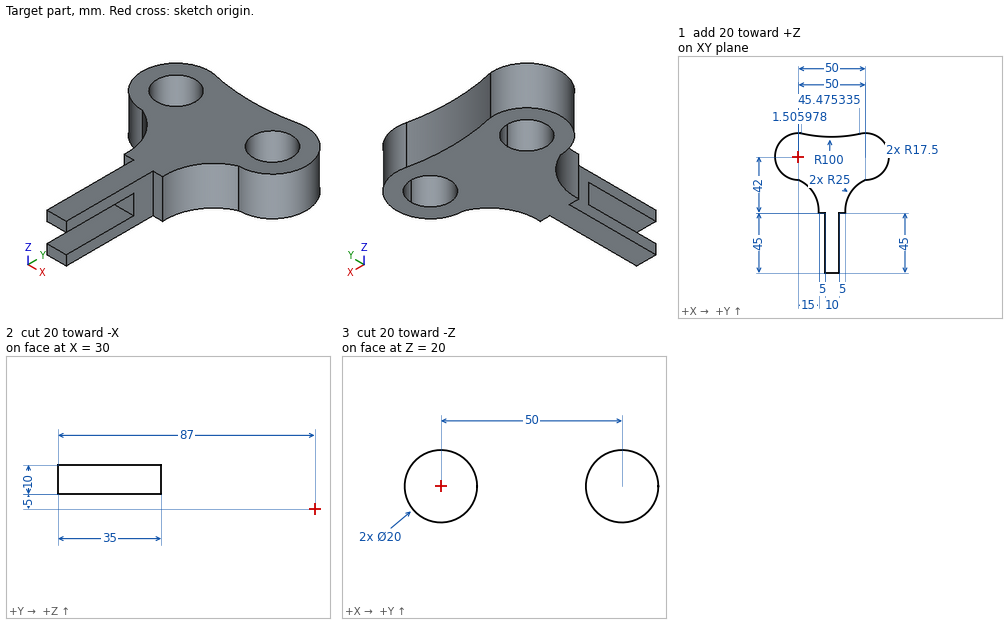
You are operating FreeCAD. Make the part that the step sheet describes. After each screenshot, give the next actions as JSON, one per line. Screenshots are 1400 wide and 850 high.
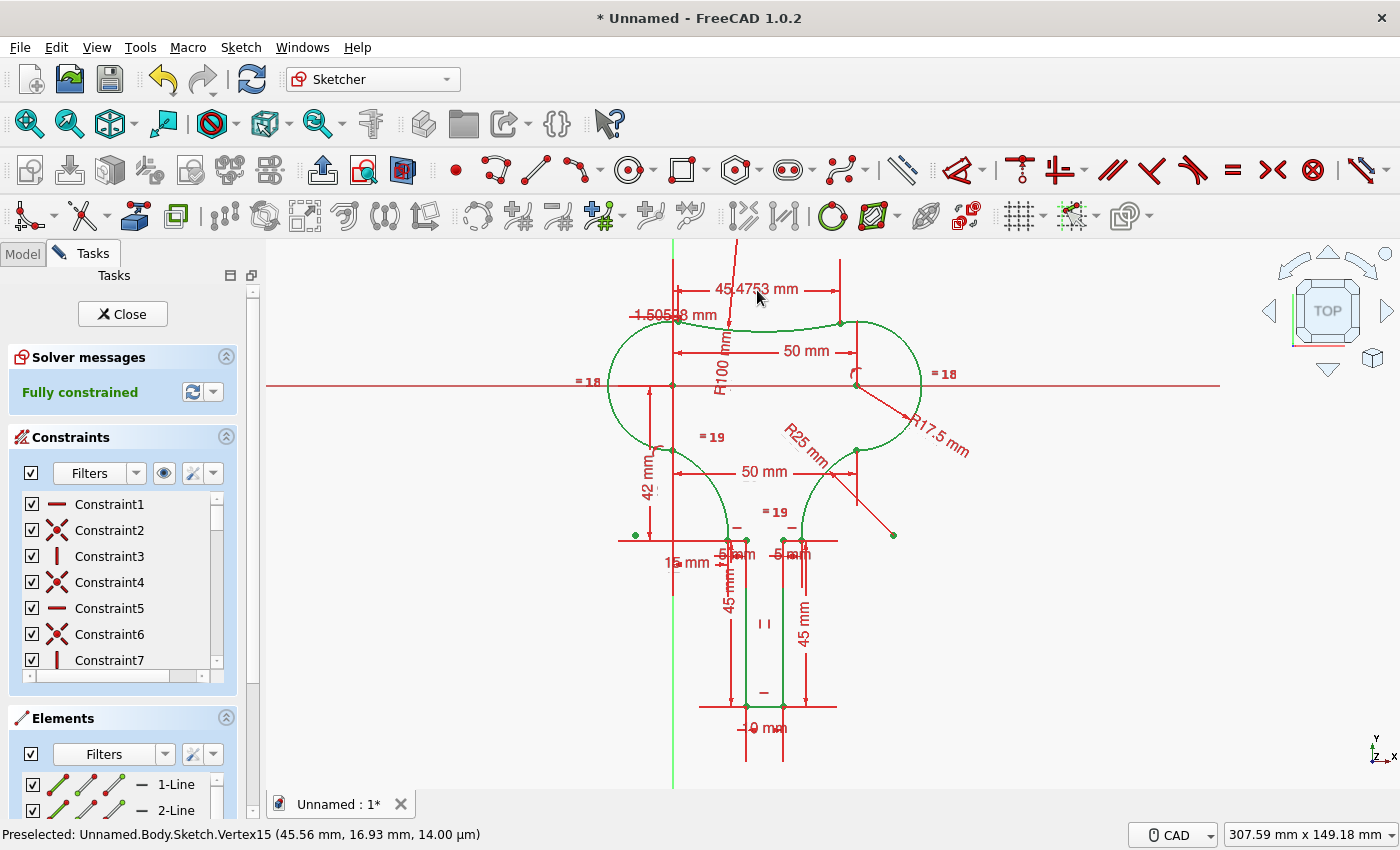
{"action": "left_click", "coordinate": [123, 314]}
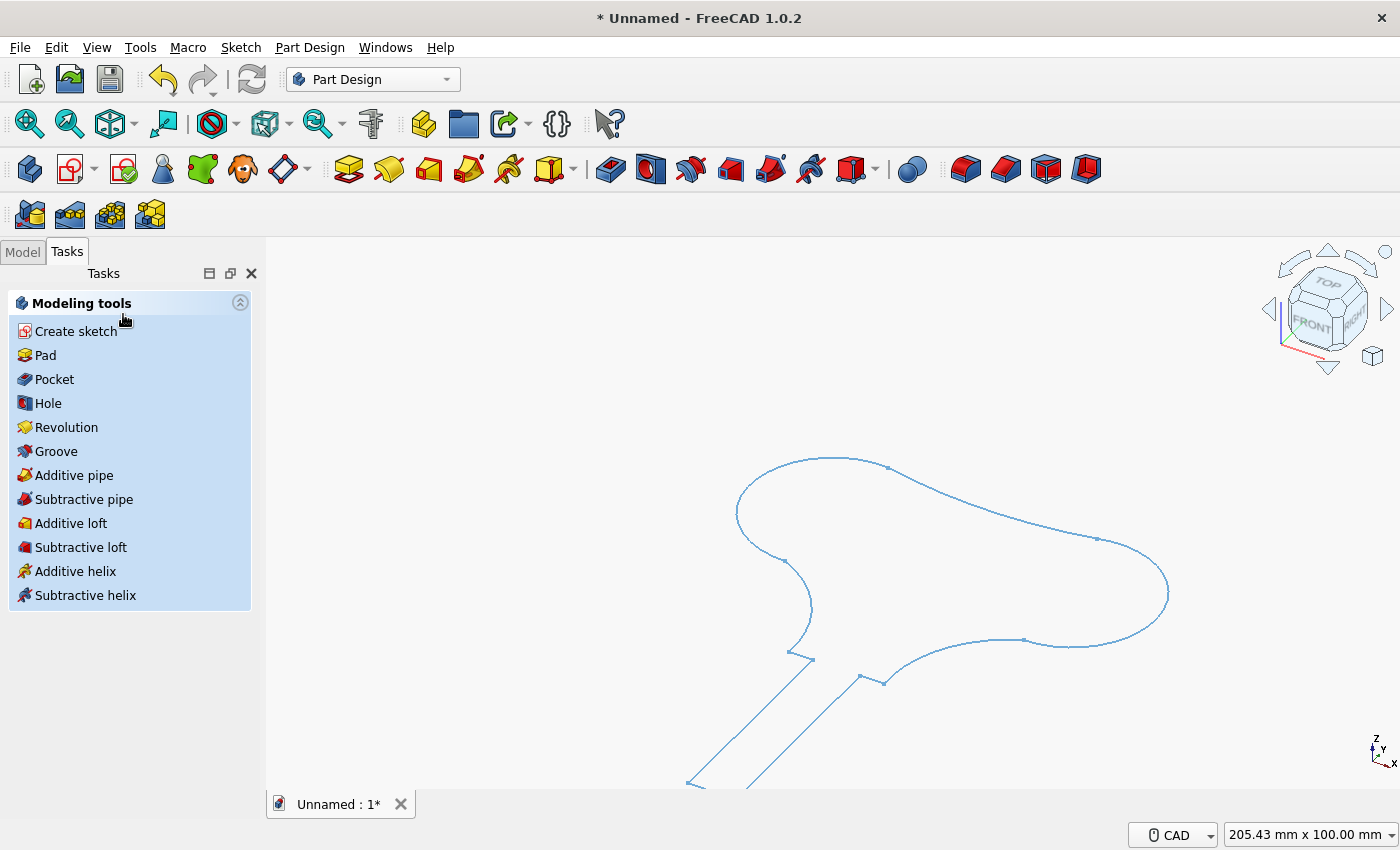
{"action": "left_click", "coordinate": [350, 170]}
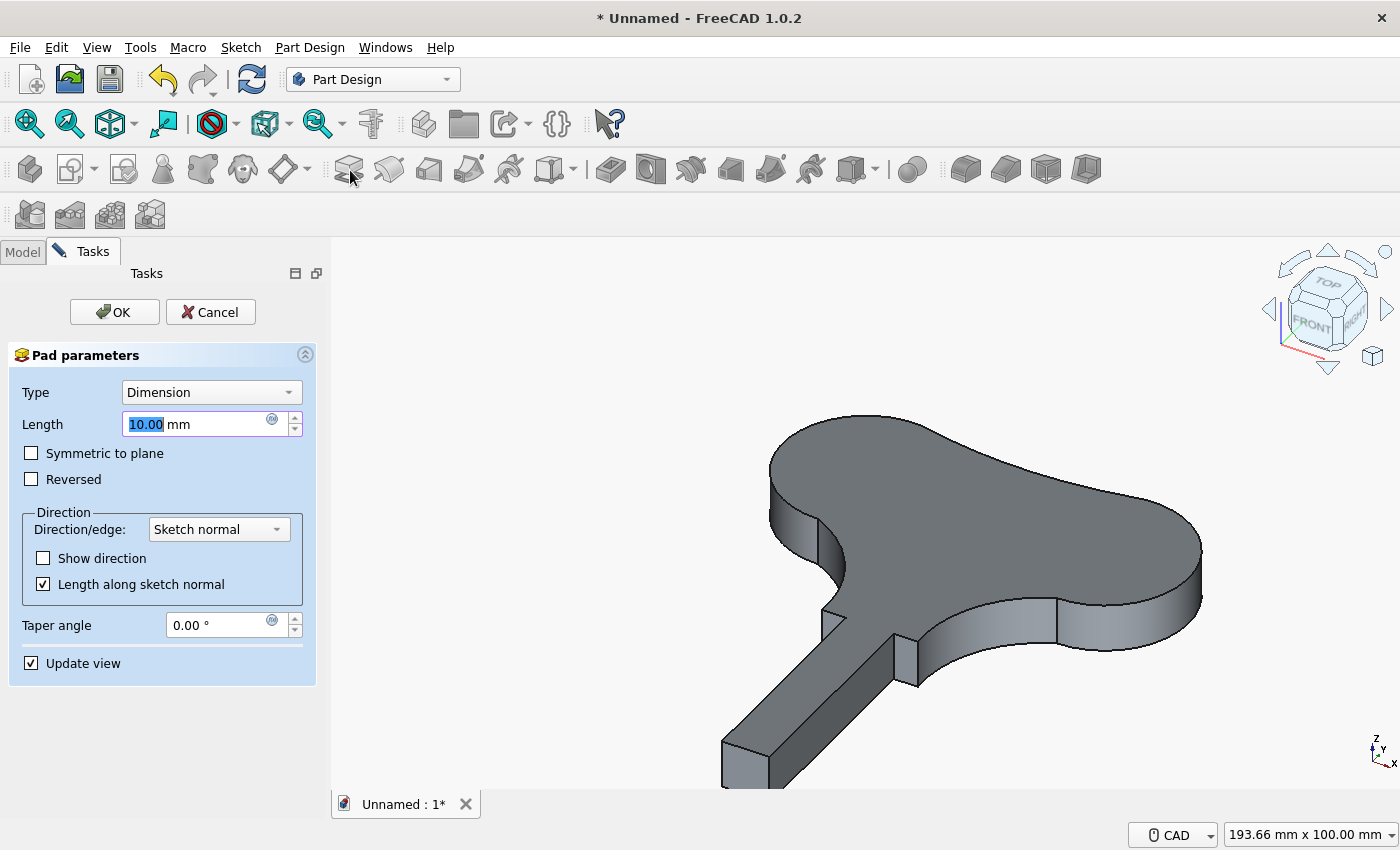
{"action": "type", "text": "20"}
{"action": "key", "text": "Tab"}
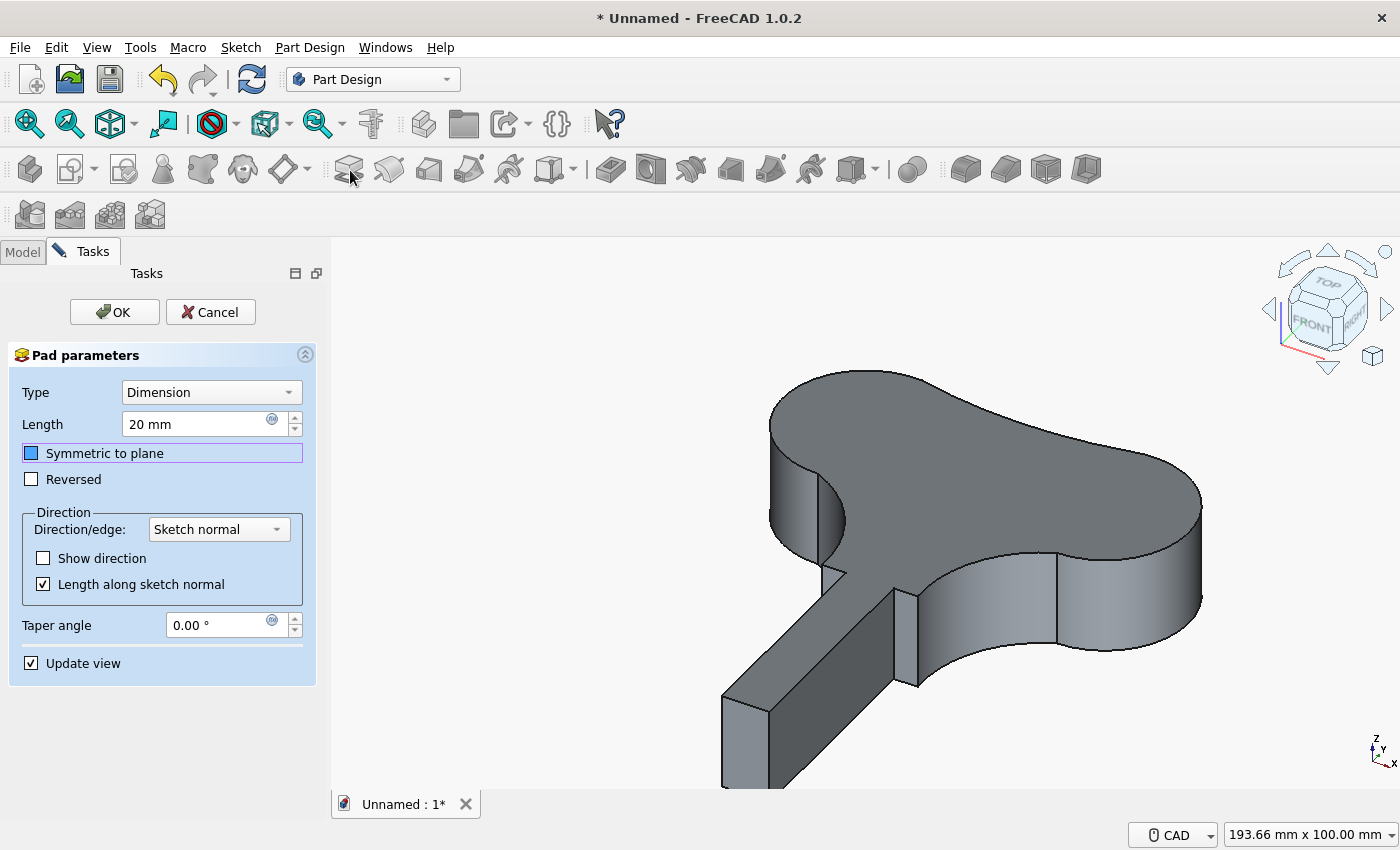
{"action": "left_click", "coordinate": [115, 312]}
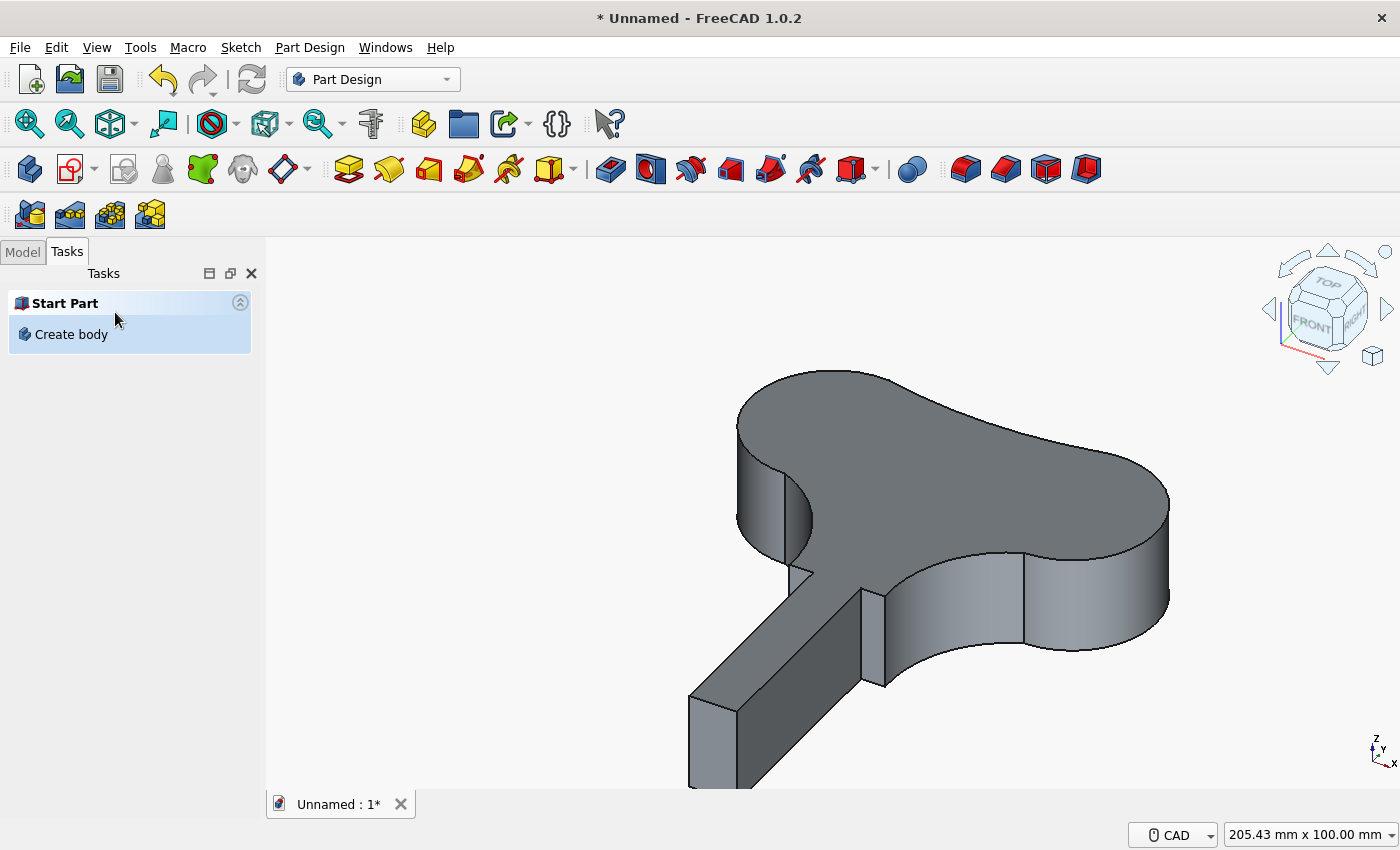
{"action": "left_click", "coordinate": [30, 124]}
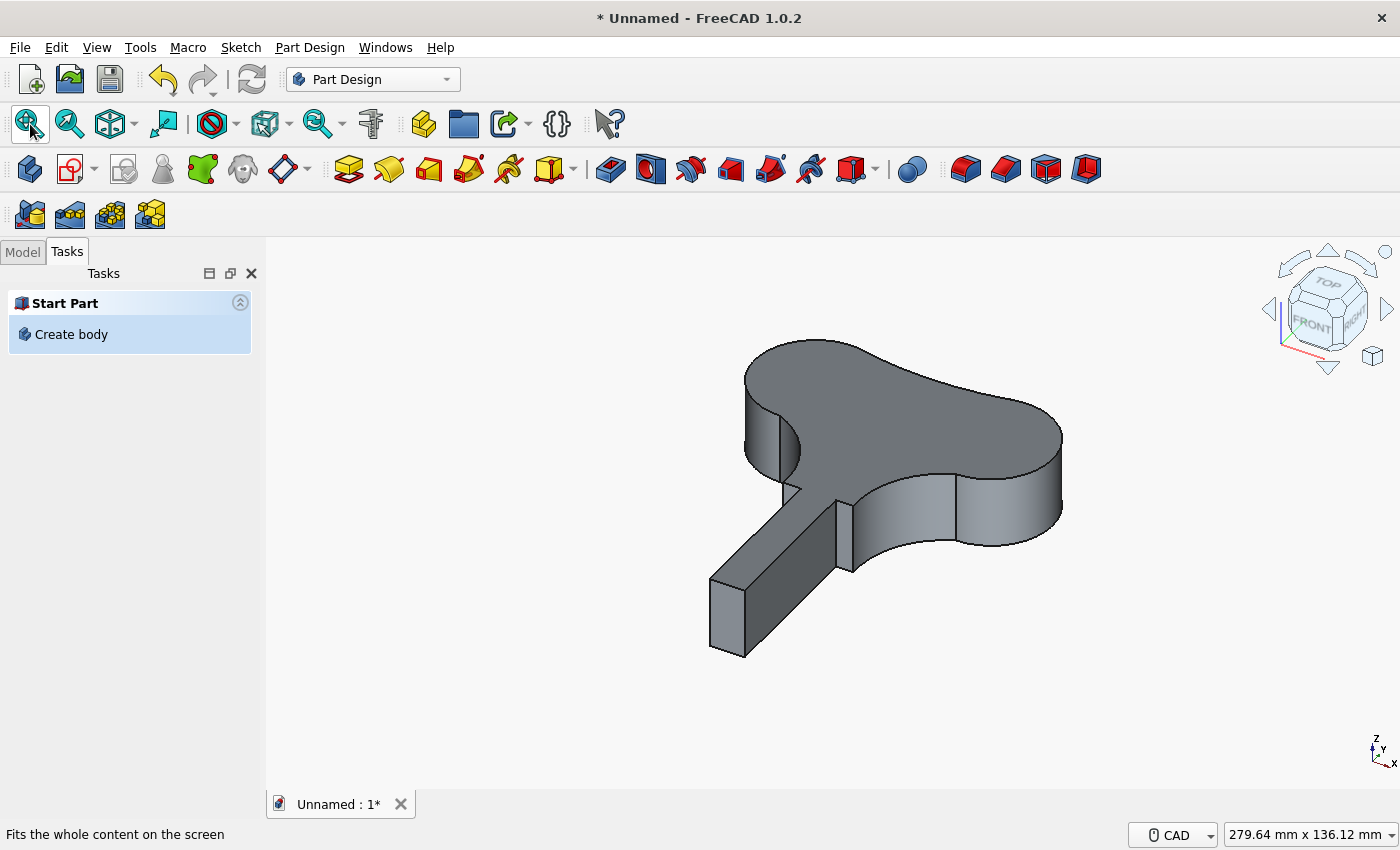
{"action": "left_click", "coordinate": [803, 565]}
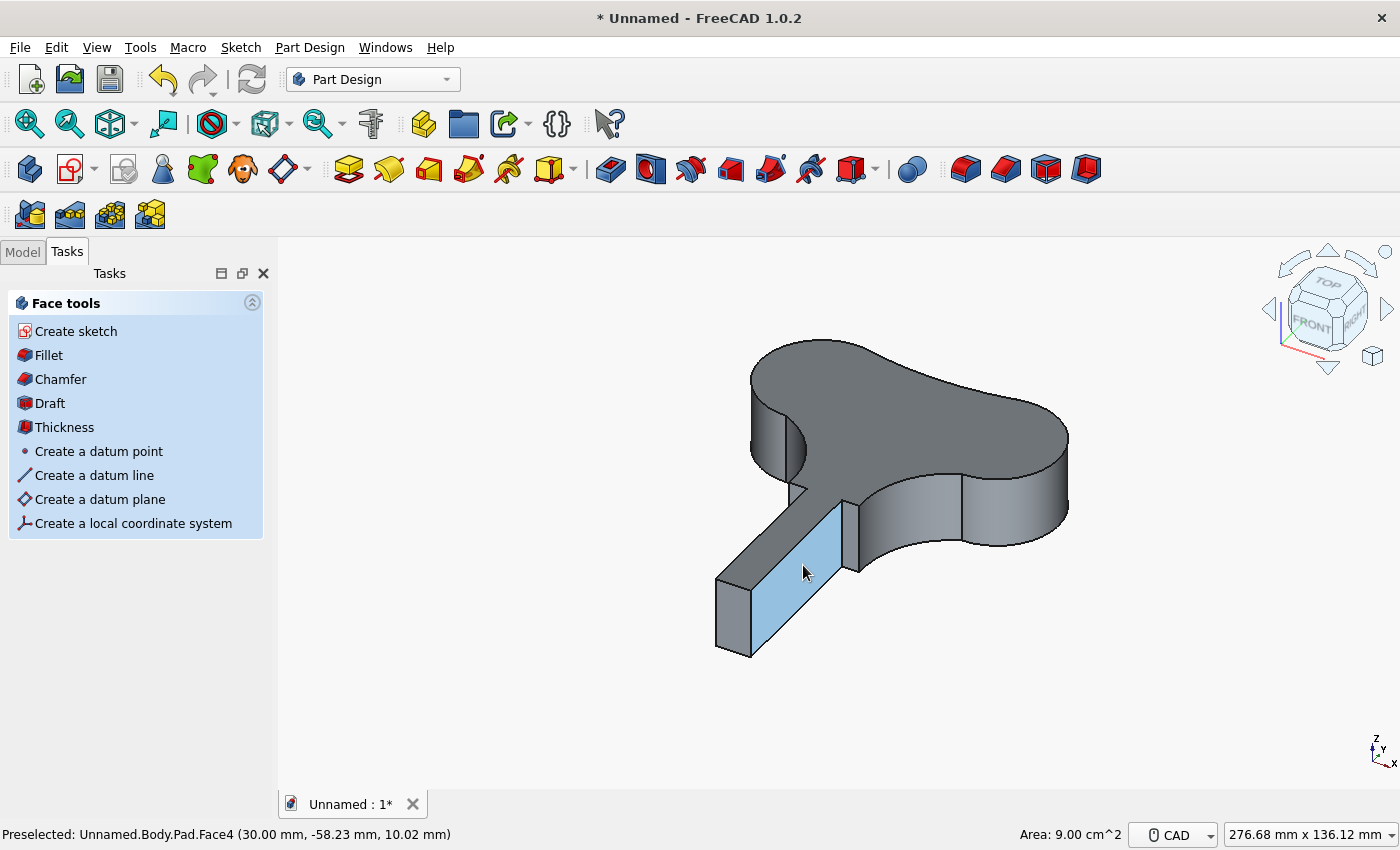
{"action": "left_click", "coordinate": [70, 170]}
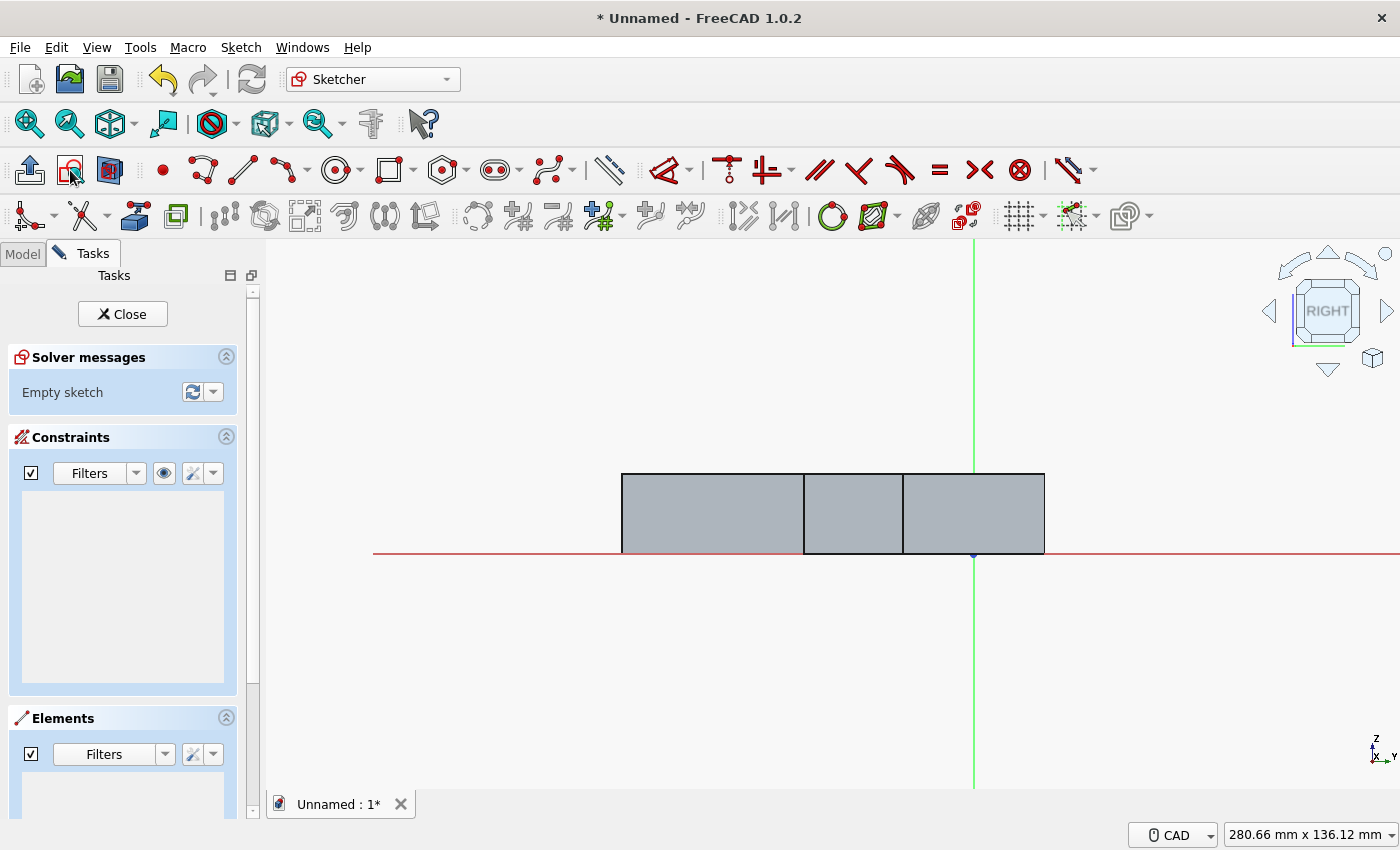
{"action": "scroll", "coordinate": [838, 536], "scroll_direction": "up", "scroll_amount": 3}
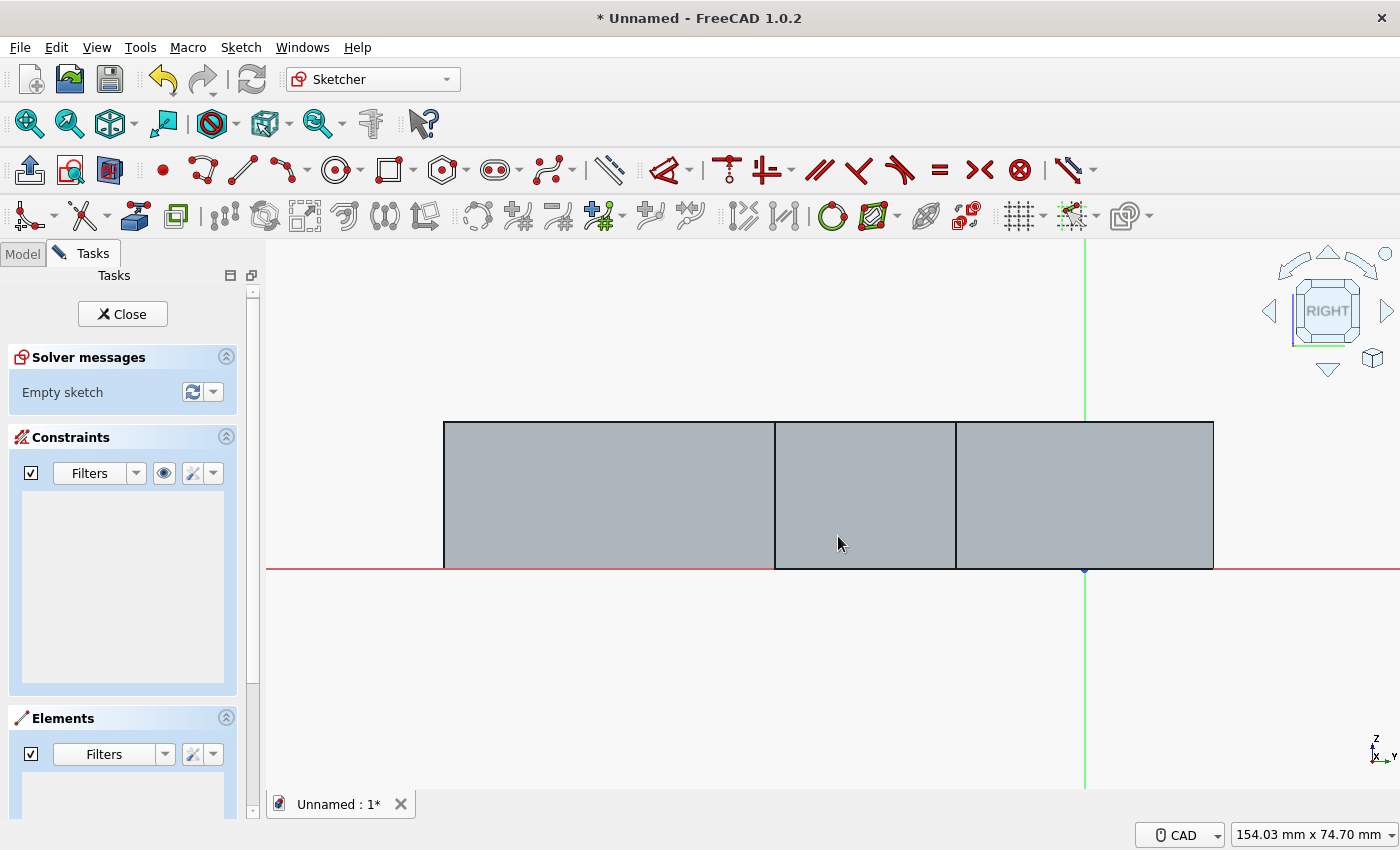
{"action": "left_click", "coordinate": [390, 170]}